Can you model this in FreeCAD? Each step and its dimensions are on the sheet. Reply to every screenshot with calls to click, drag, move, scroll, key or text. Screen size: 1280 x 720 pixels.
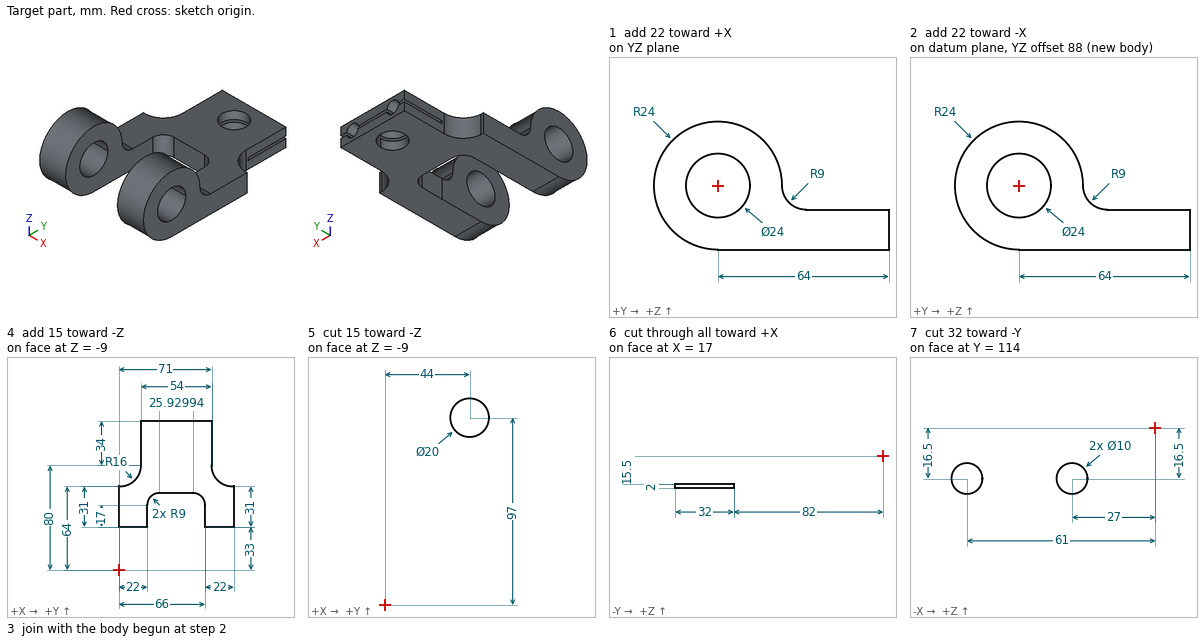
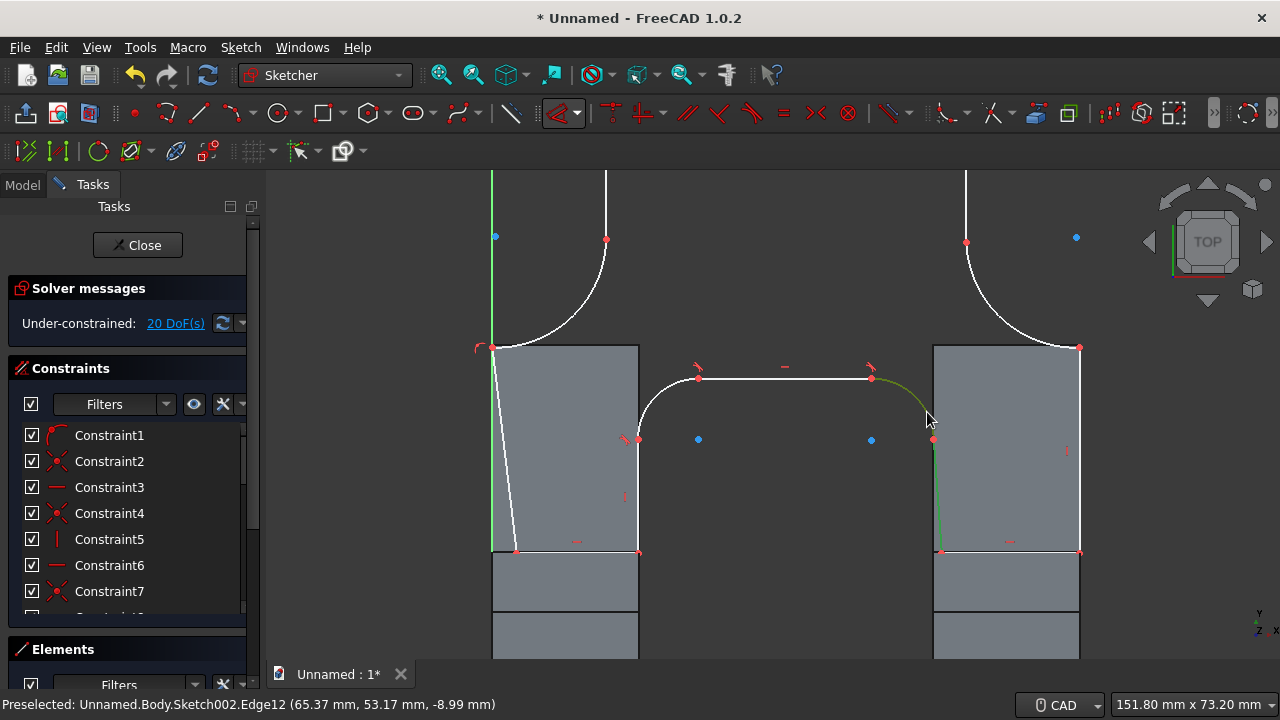
click(752, 114)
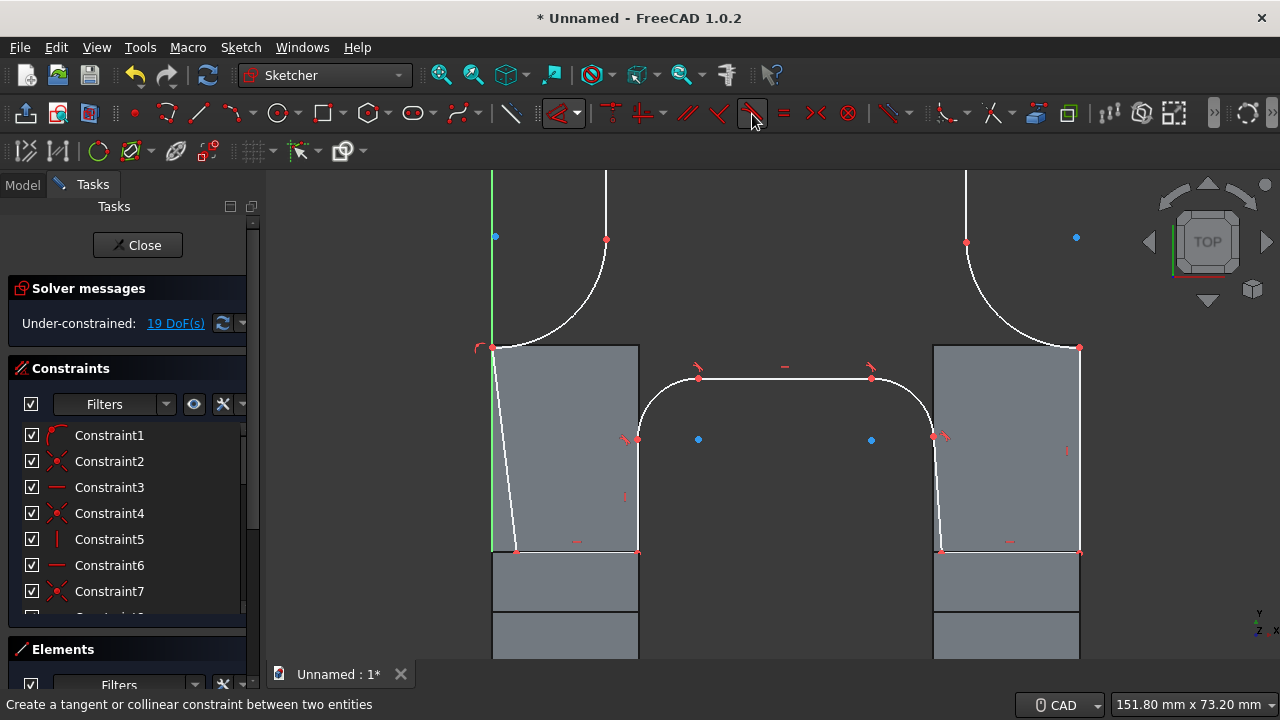
scroll(657, 428, down, 5)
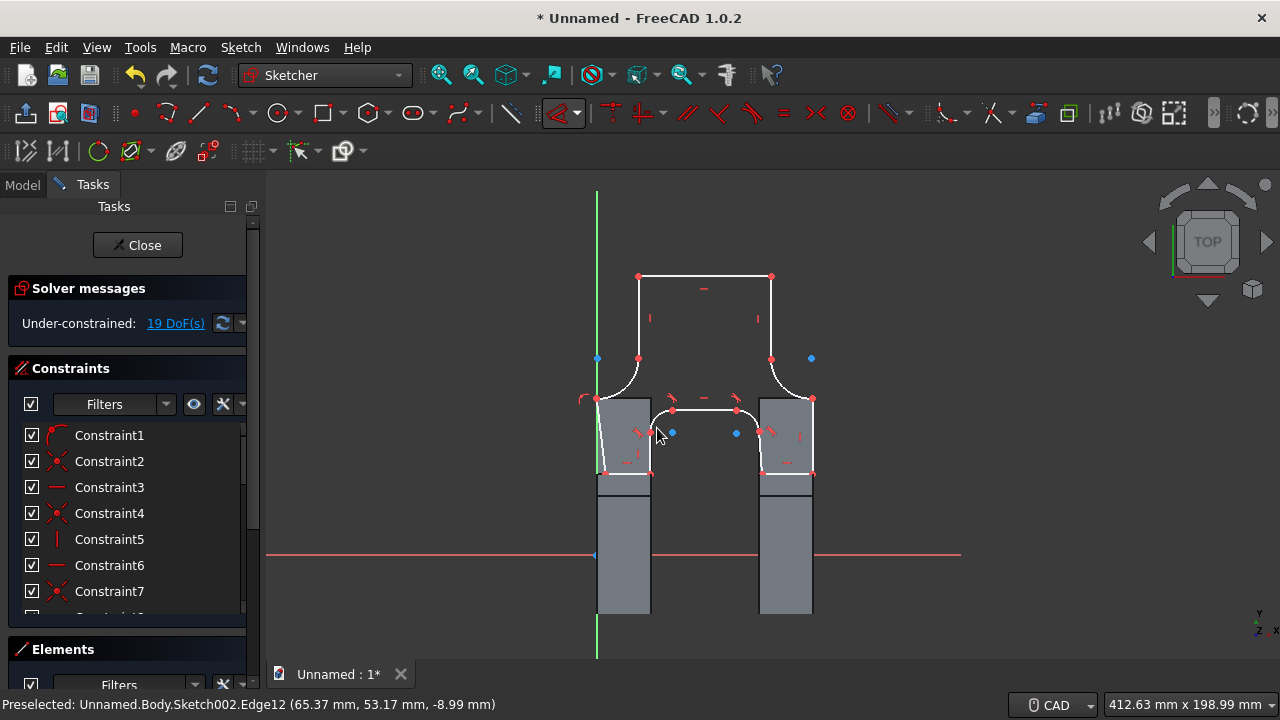
click(771, 335)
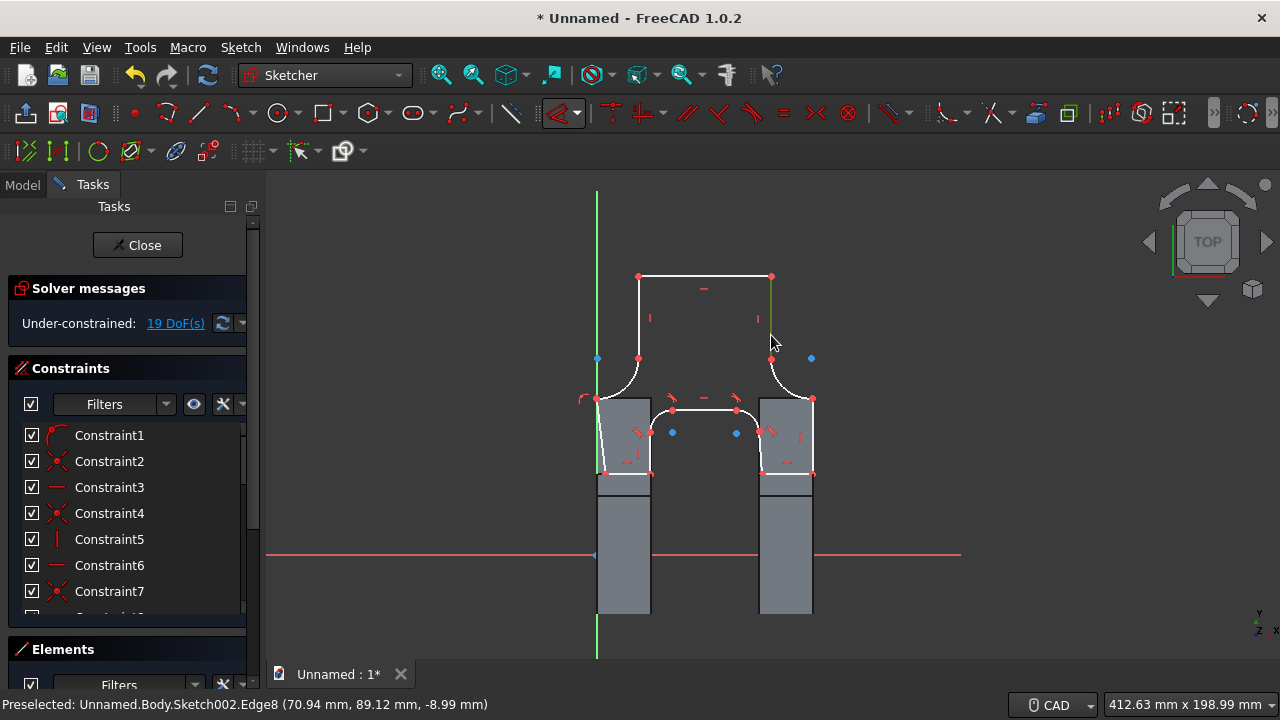
click(776, 378)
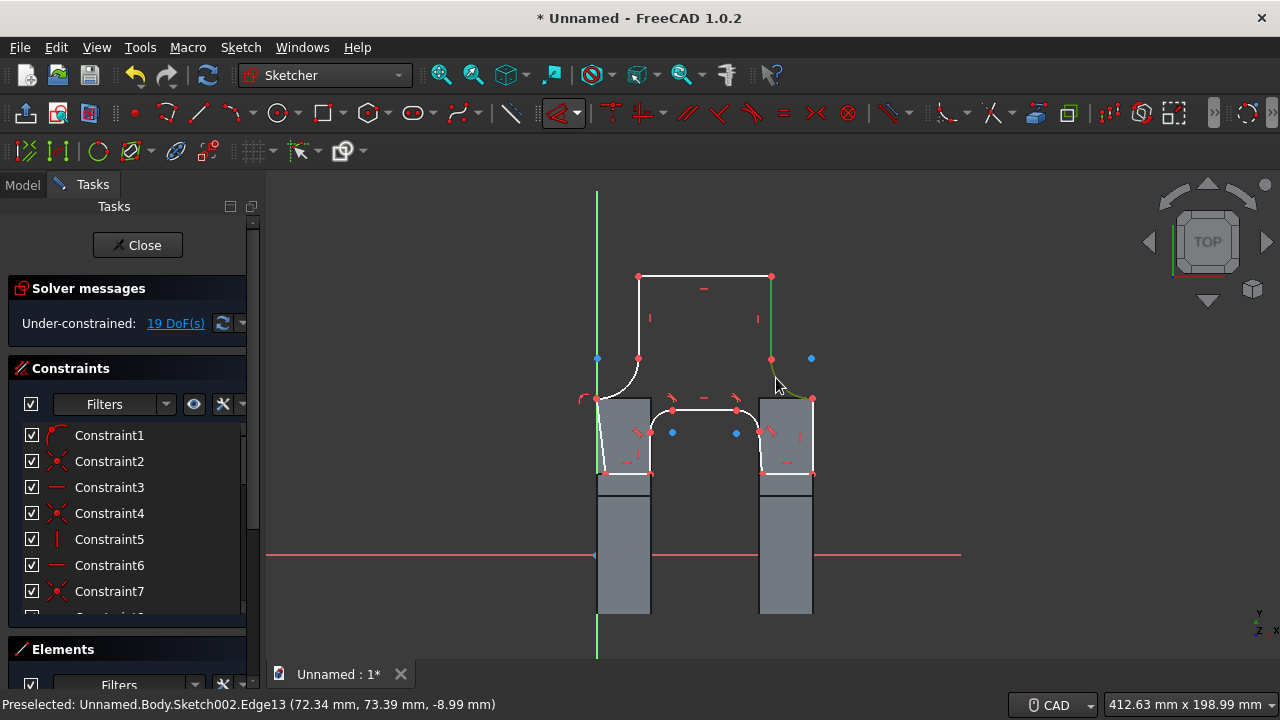
click(752, 114)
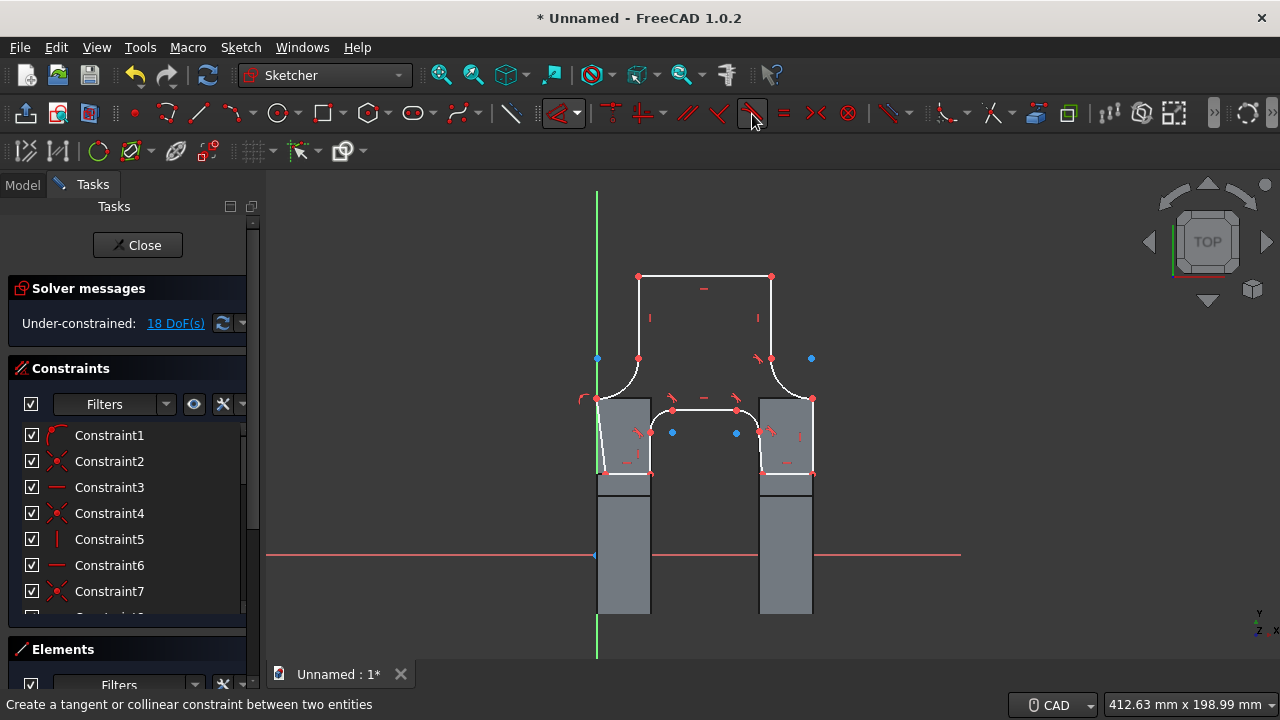
click(599, 421)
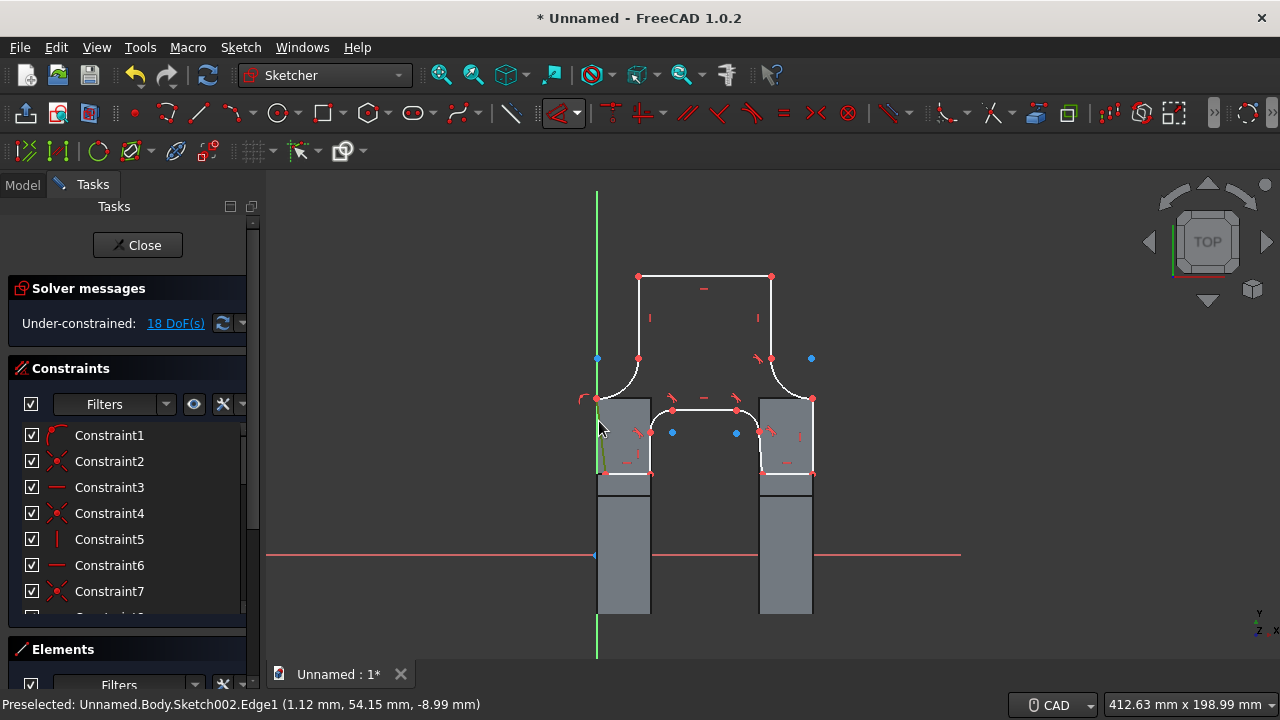
click(666, 114)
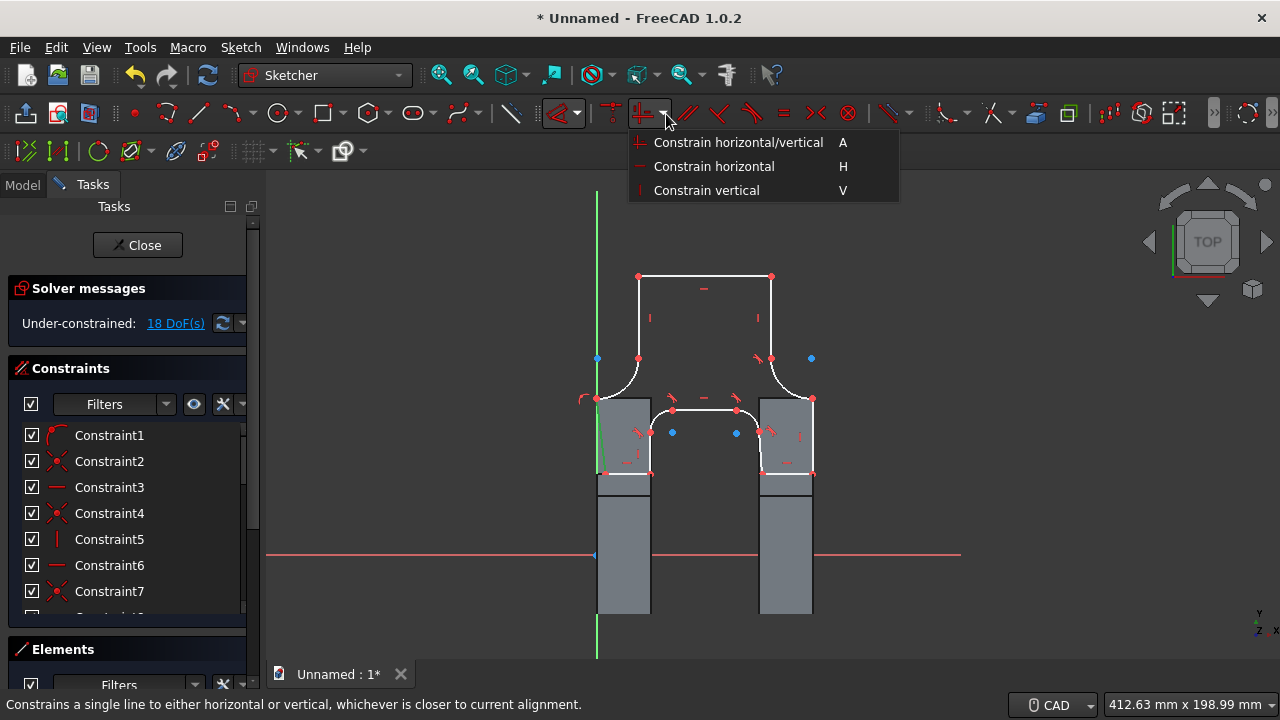
click(764, 190)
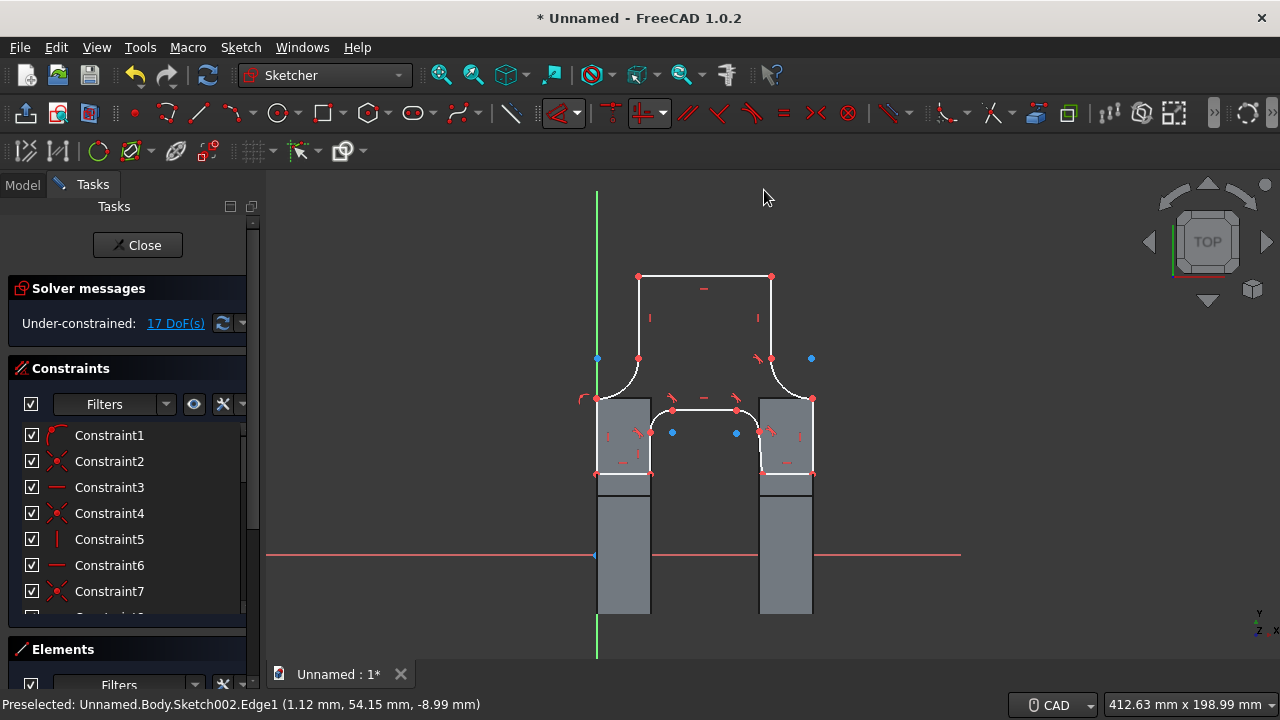
scroll(662, 413, up, 2)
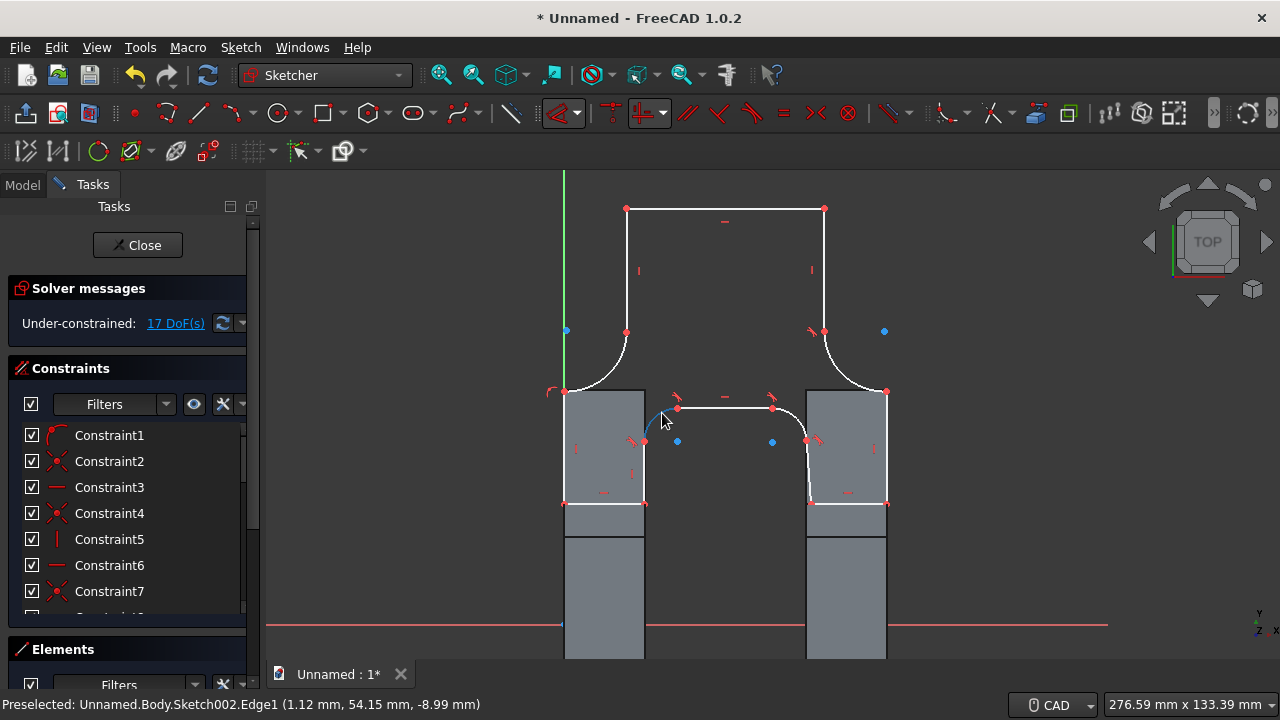
click(662, 412)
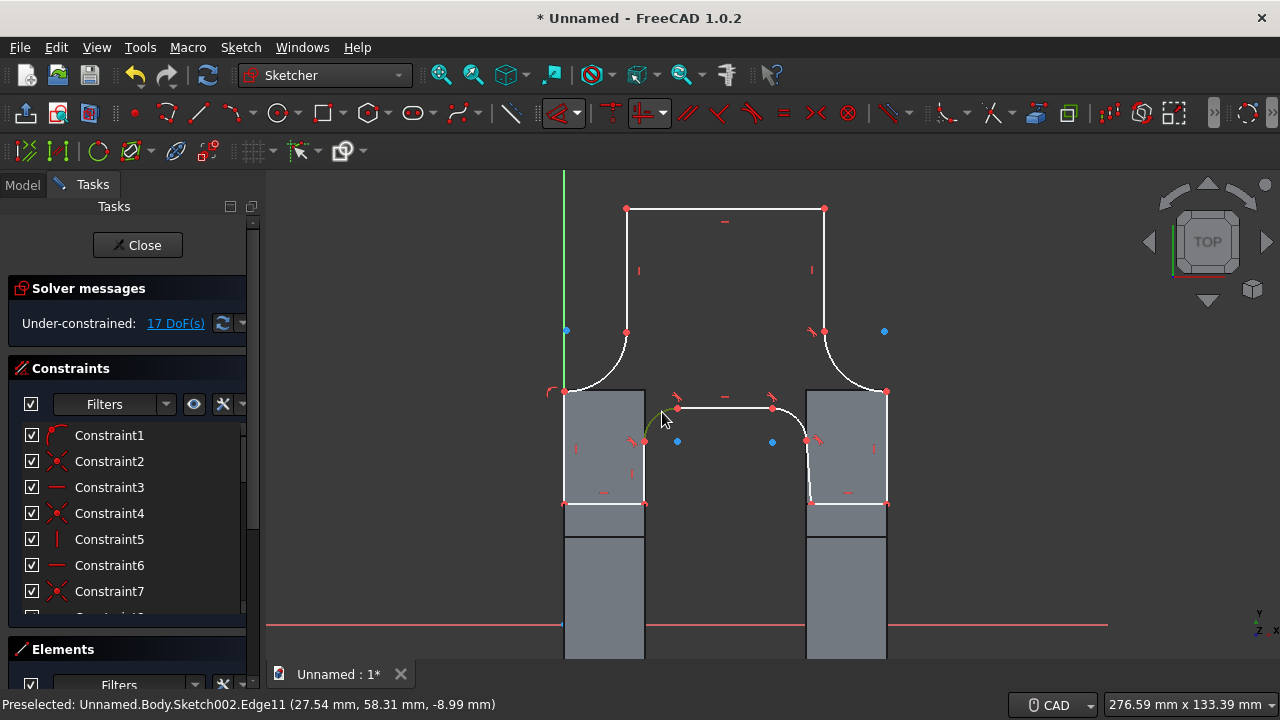
click(802, 426)